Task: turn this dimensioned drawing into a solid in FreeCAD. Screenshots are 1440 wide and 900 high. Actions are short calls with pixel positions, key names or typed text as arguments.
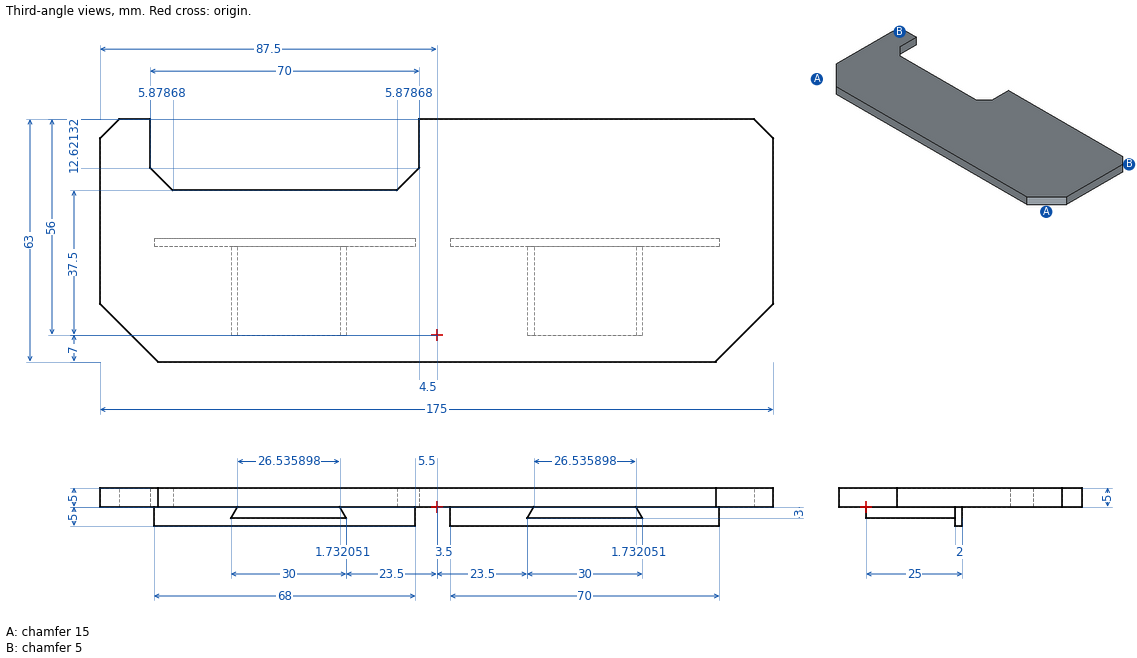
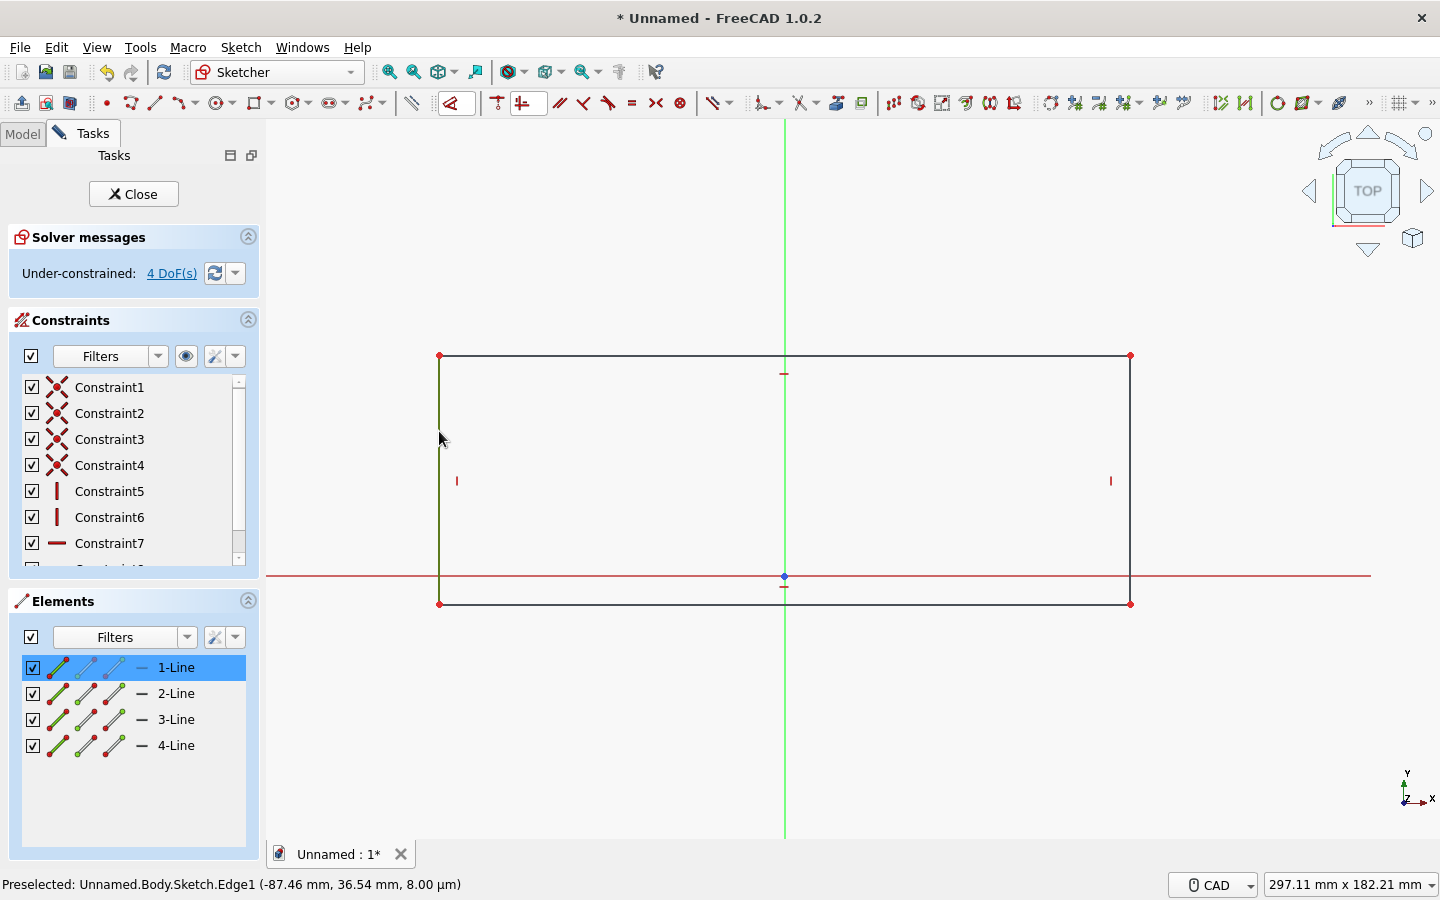
key(i)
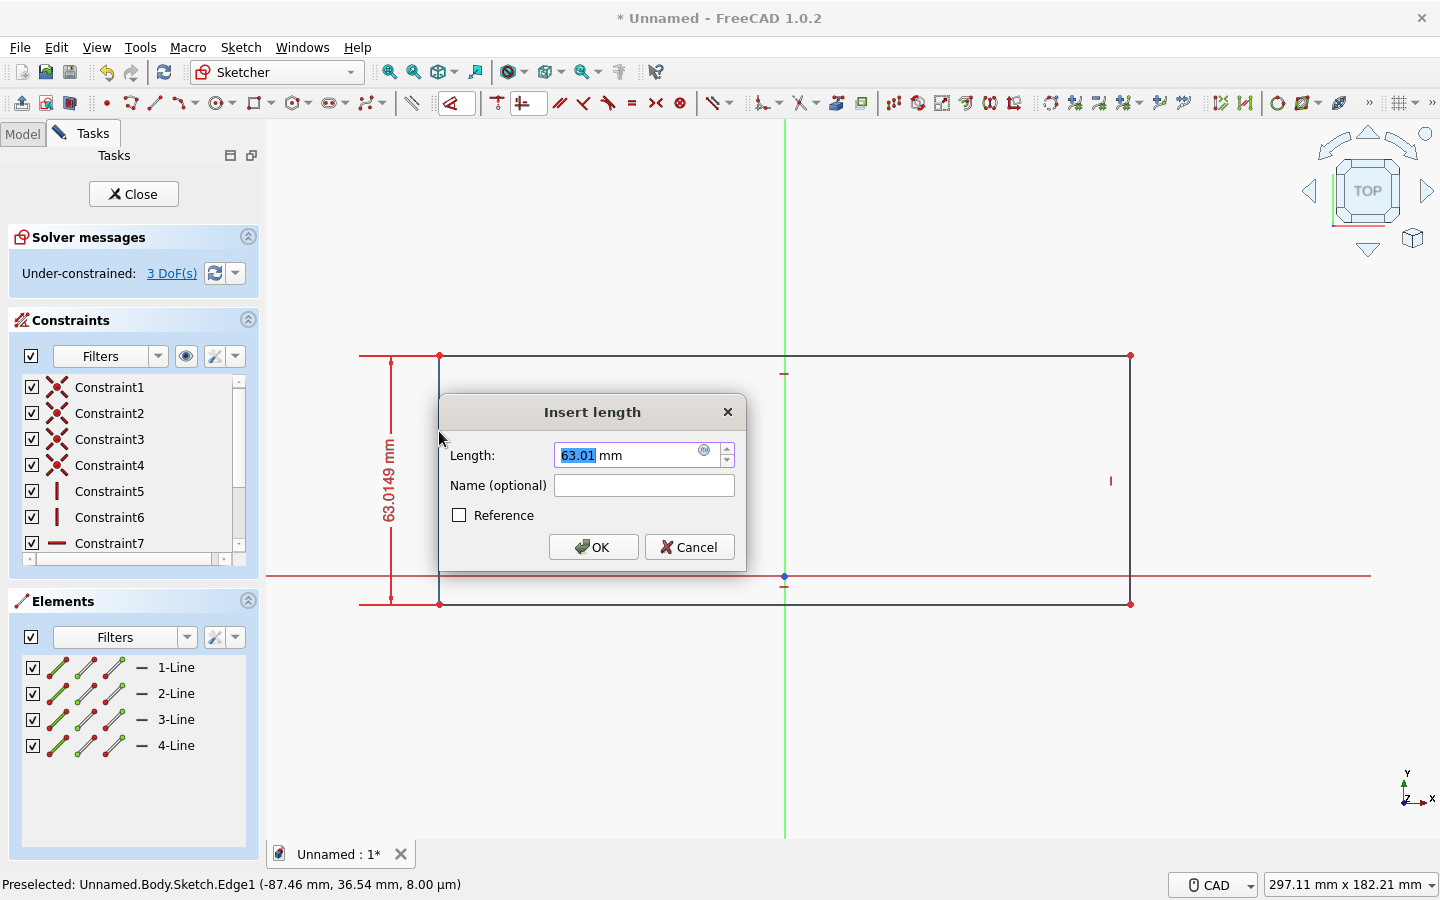
text(63)
key(Return)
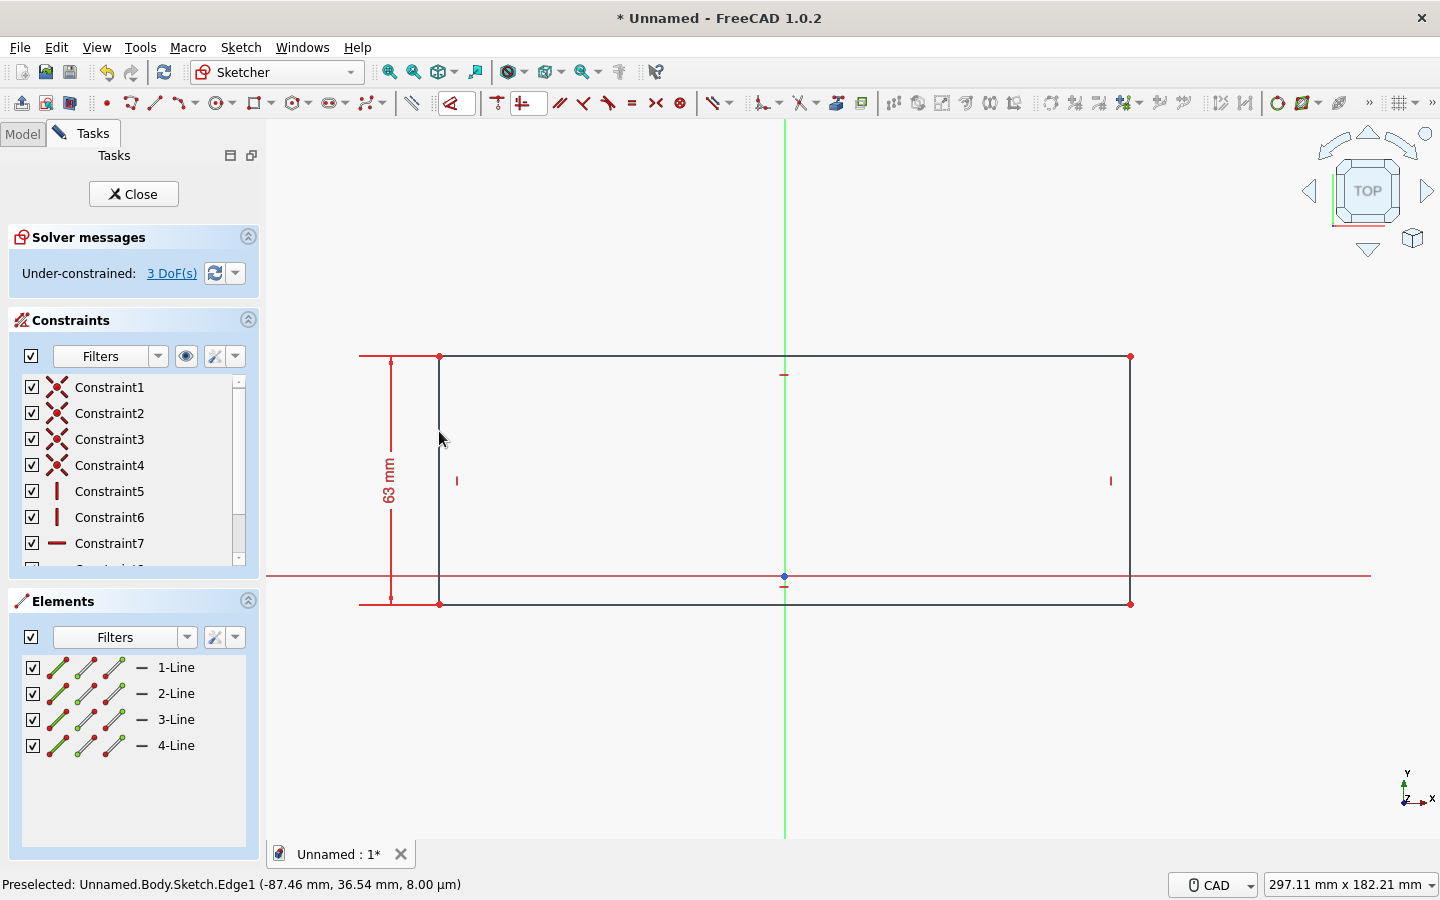
scroll(439, 605, up, 2)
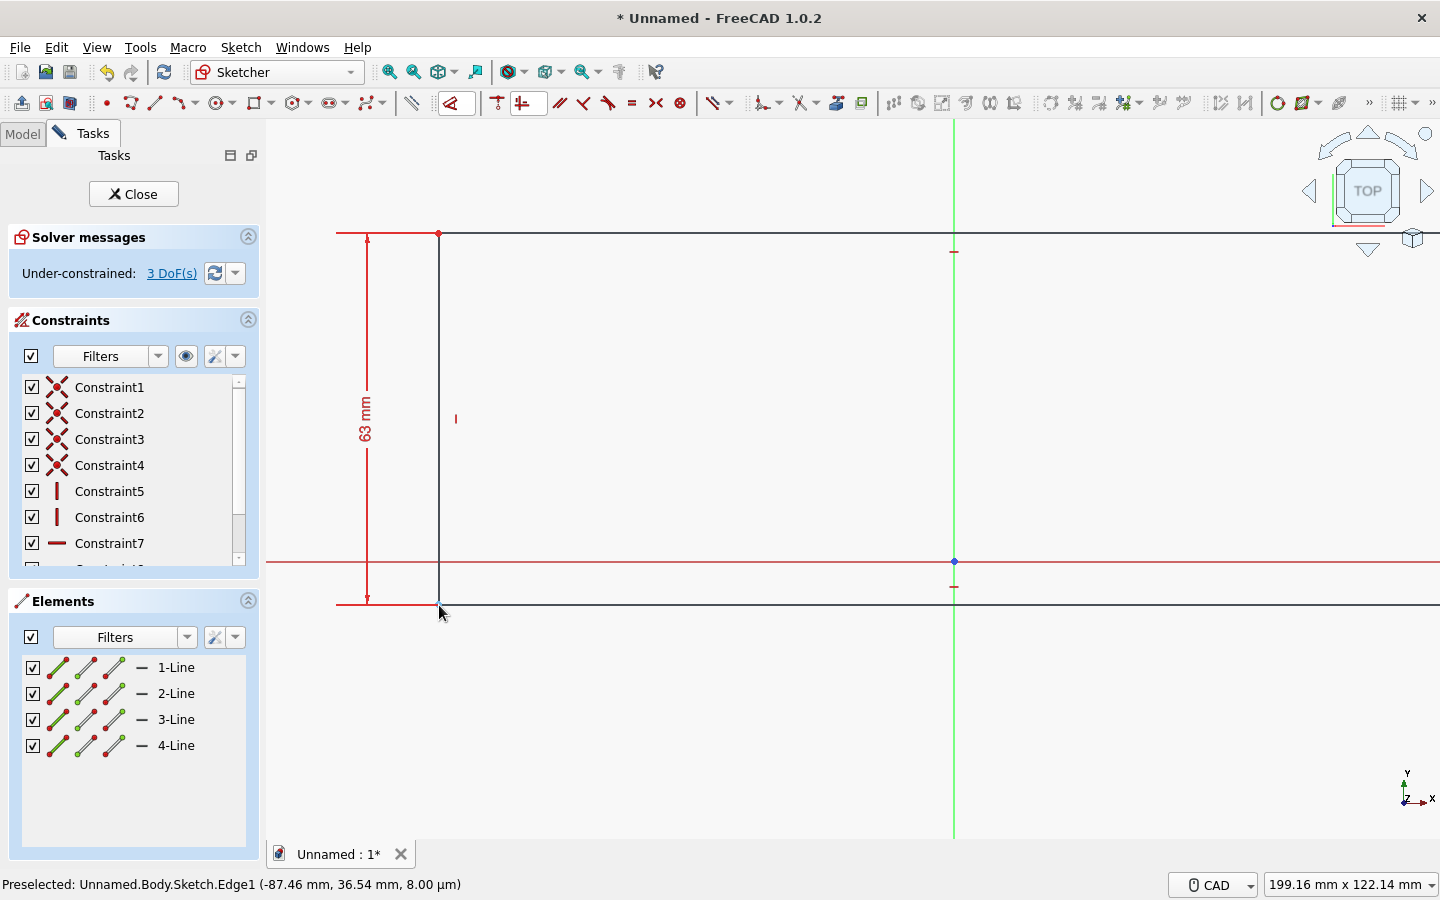
click(439, 605)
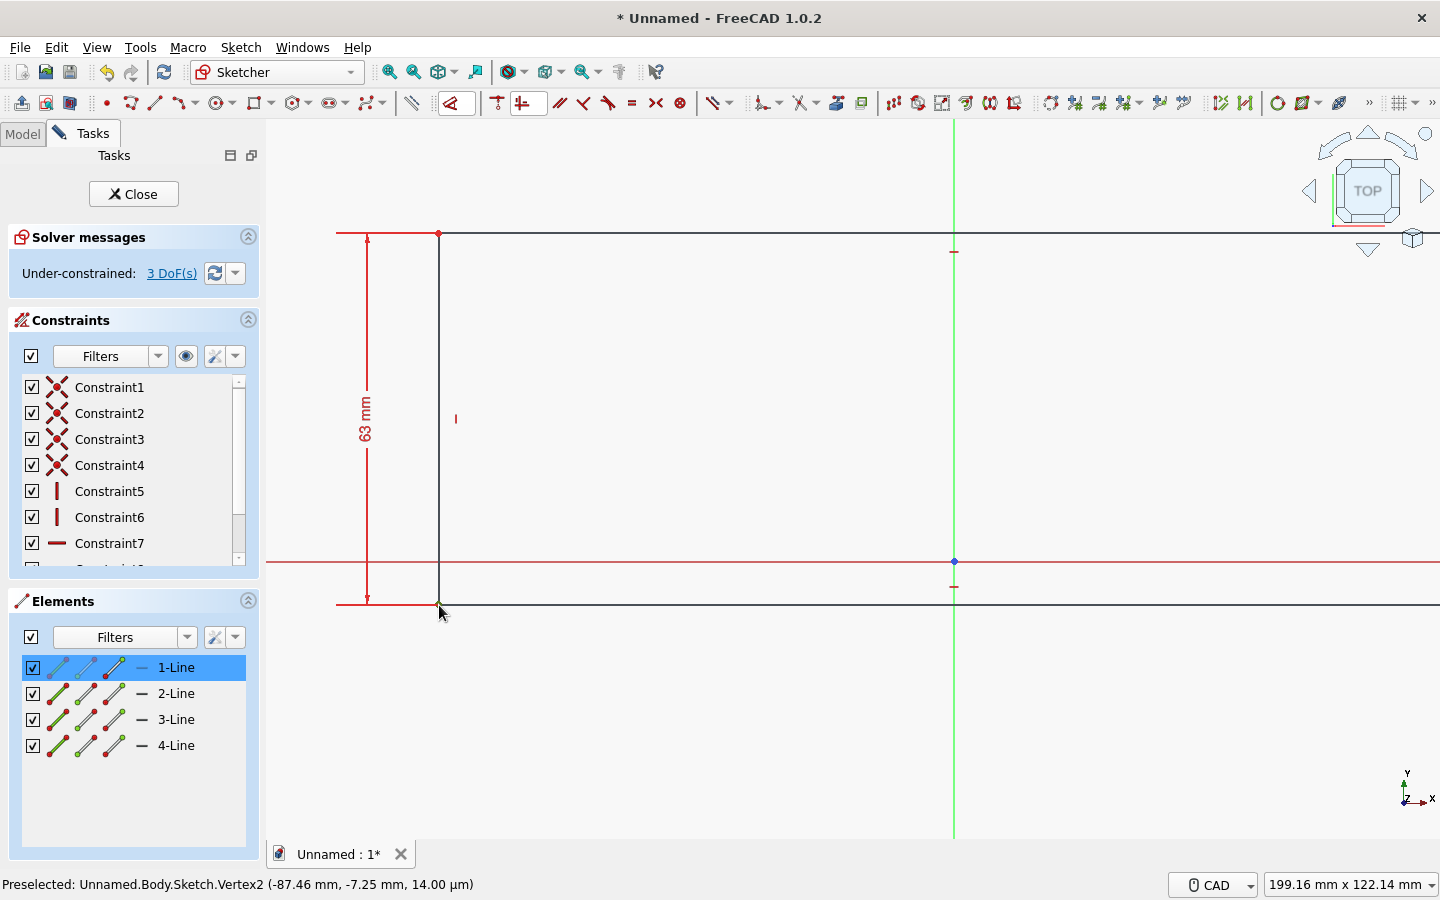
click(470, 104)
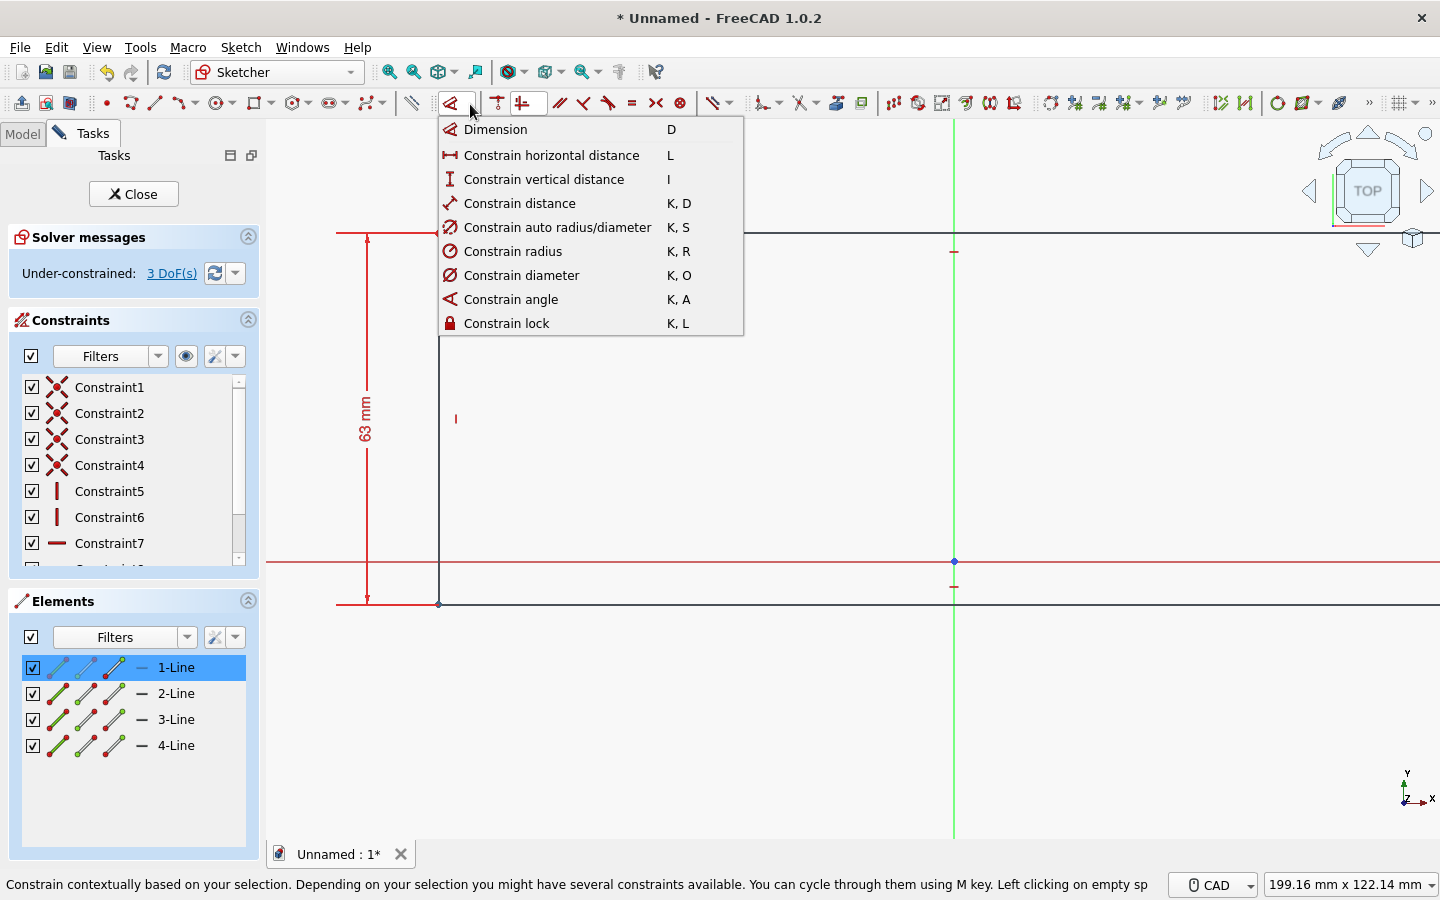
click(591, 179)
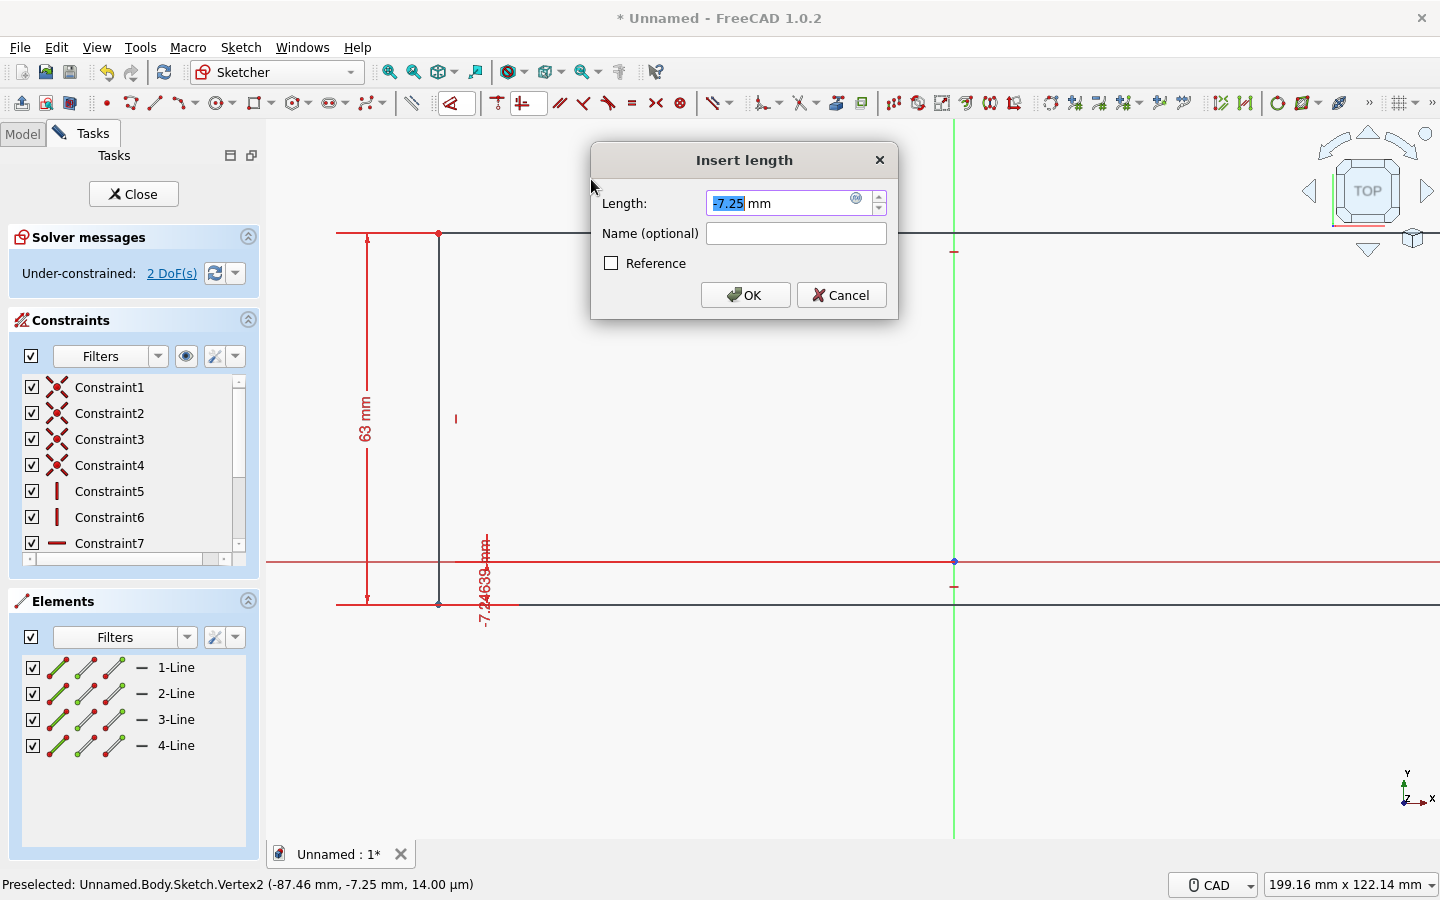
text(-7)
key(Return)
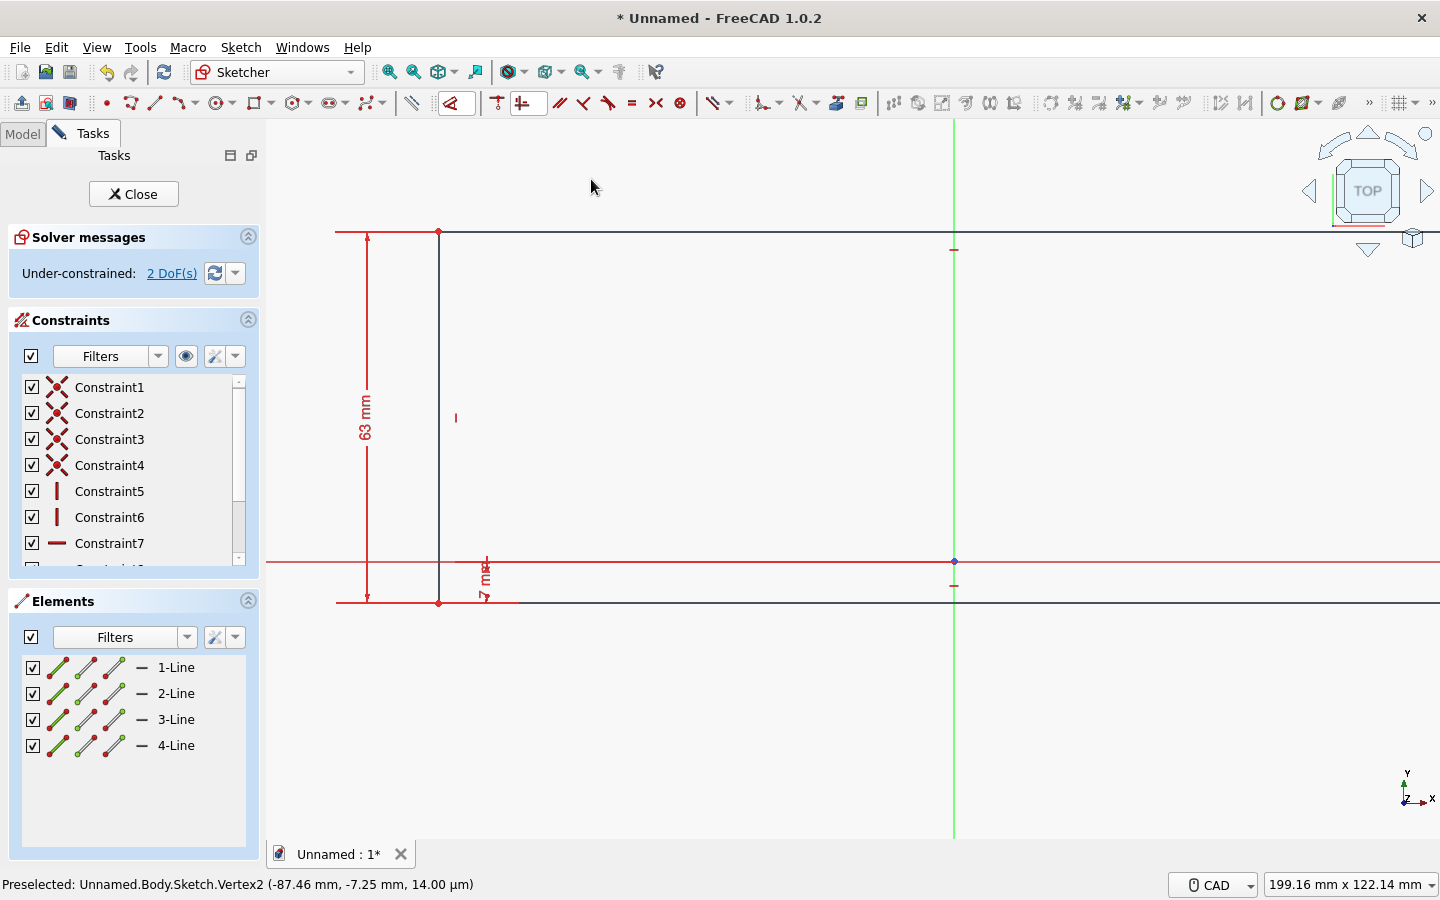
click(748, 603)